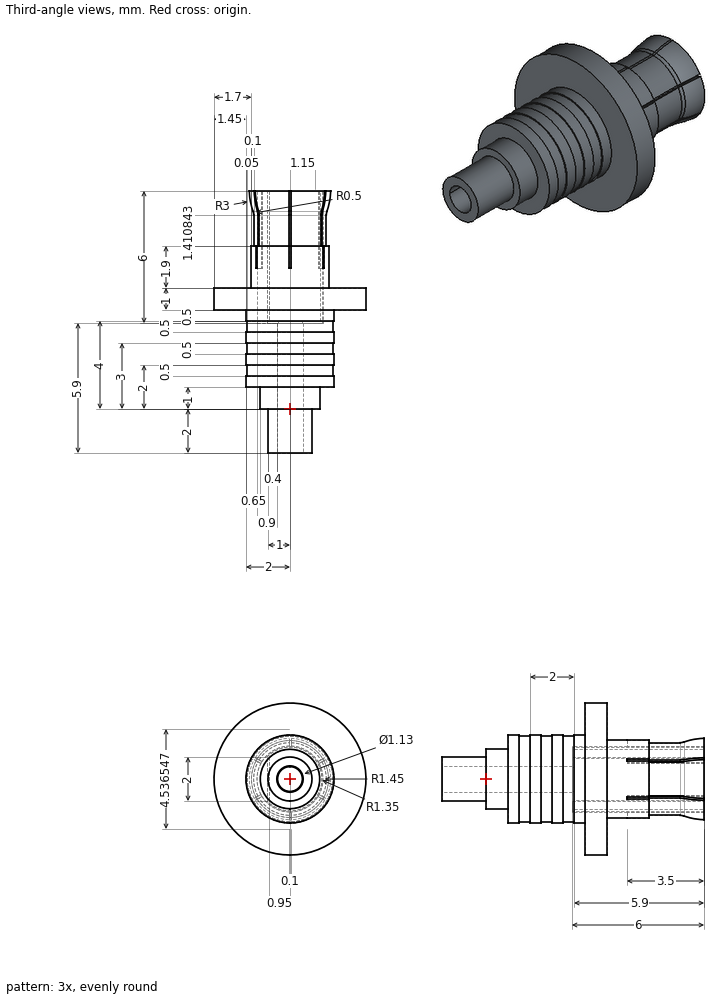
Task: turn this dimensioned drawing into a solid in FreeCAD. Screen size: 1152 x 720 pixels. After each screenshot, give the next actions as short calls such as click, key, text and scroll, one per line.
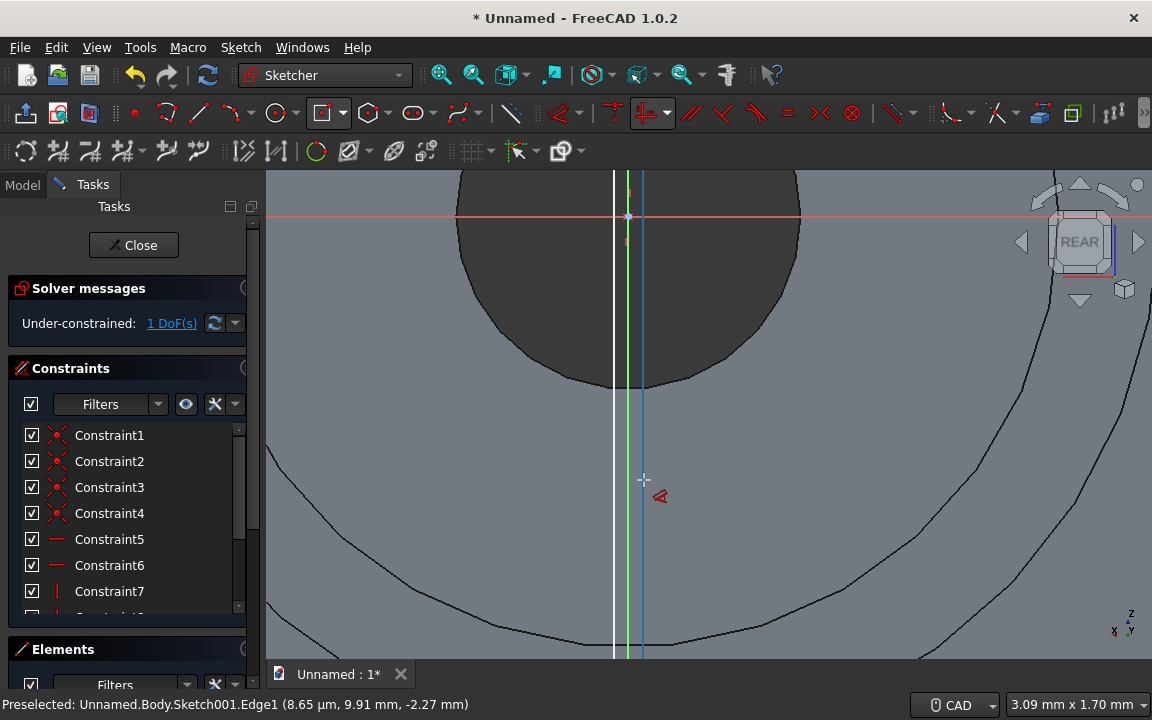
click(643, 477)
click(677, 414)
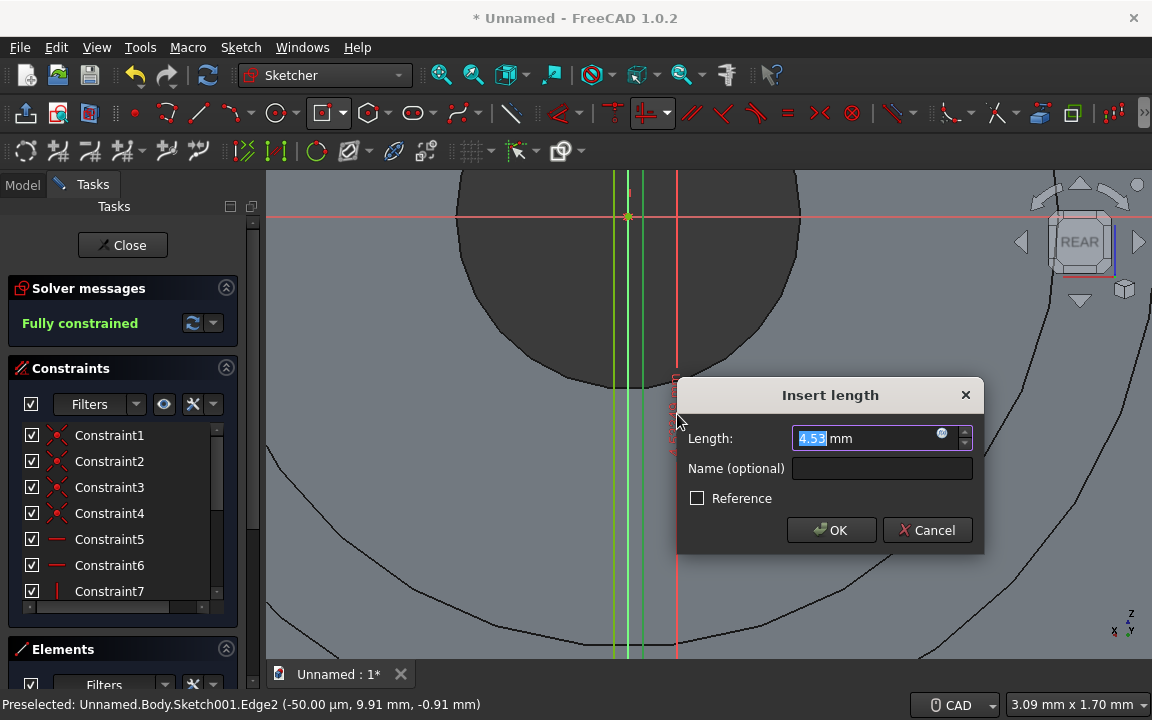
text(4.536547)
key(Return)
key(Escape)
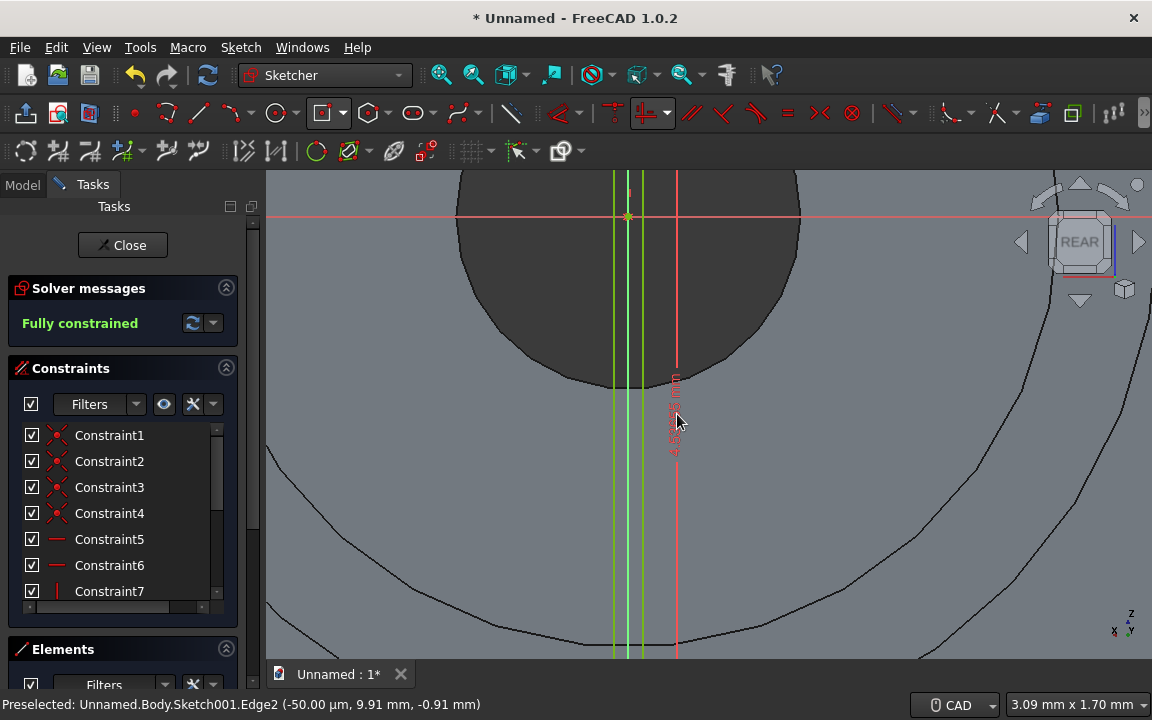
click(123, 245)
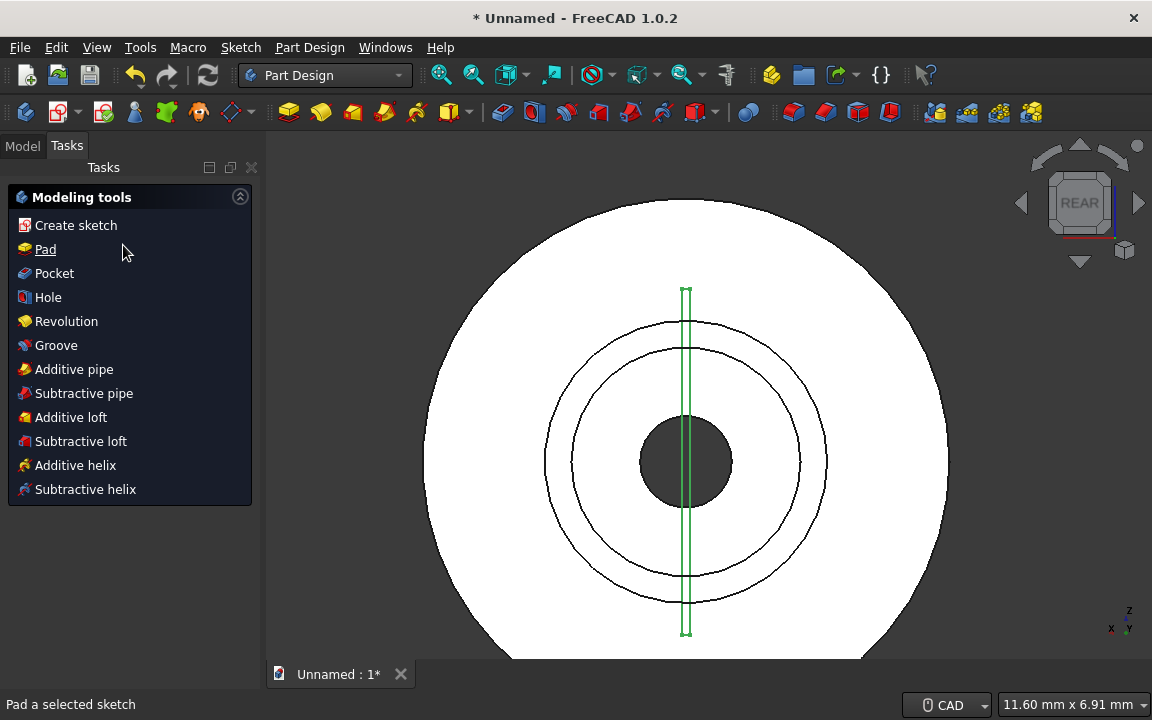
click(504, 112)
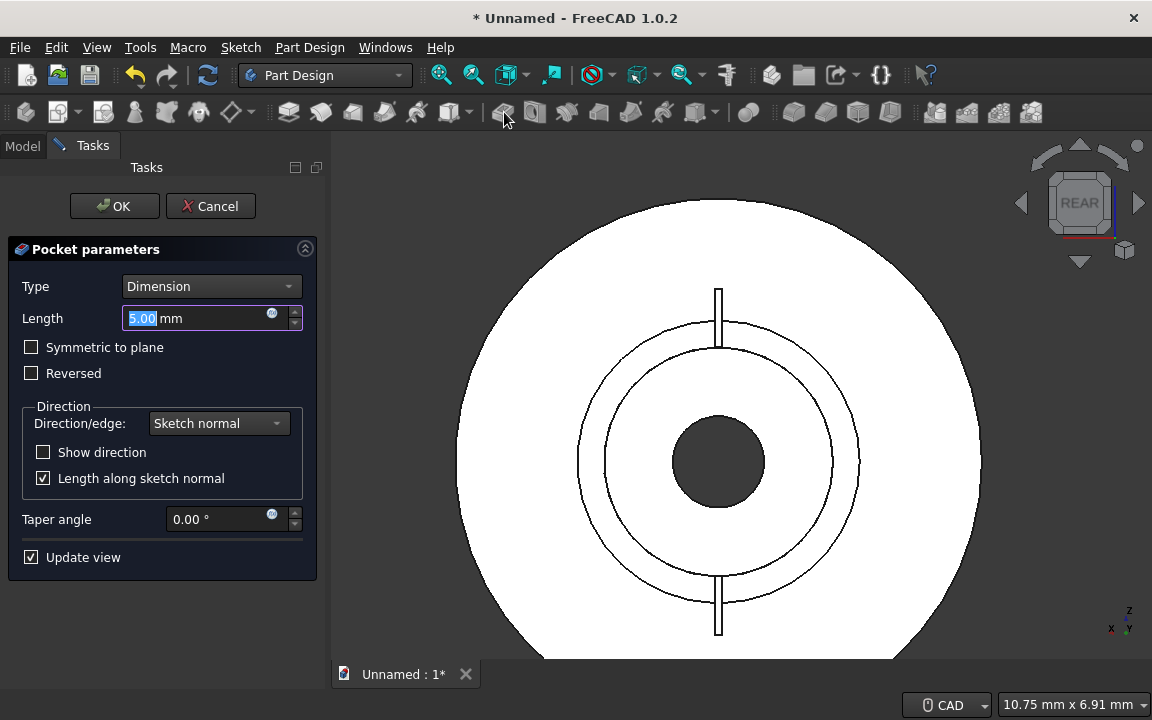
text(3.5)
key(Tab)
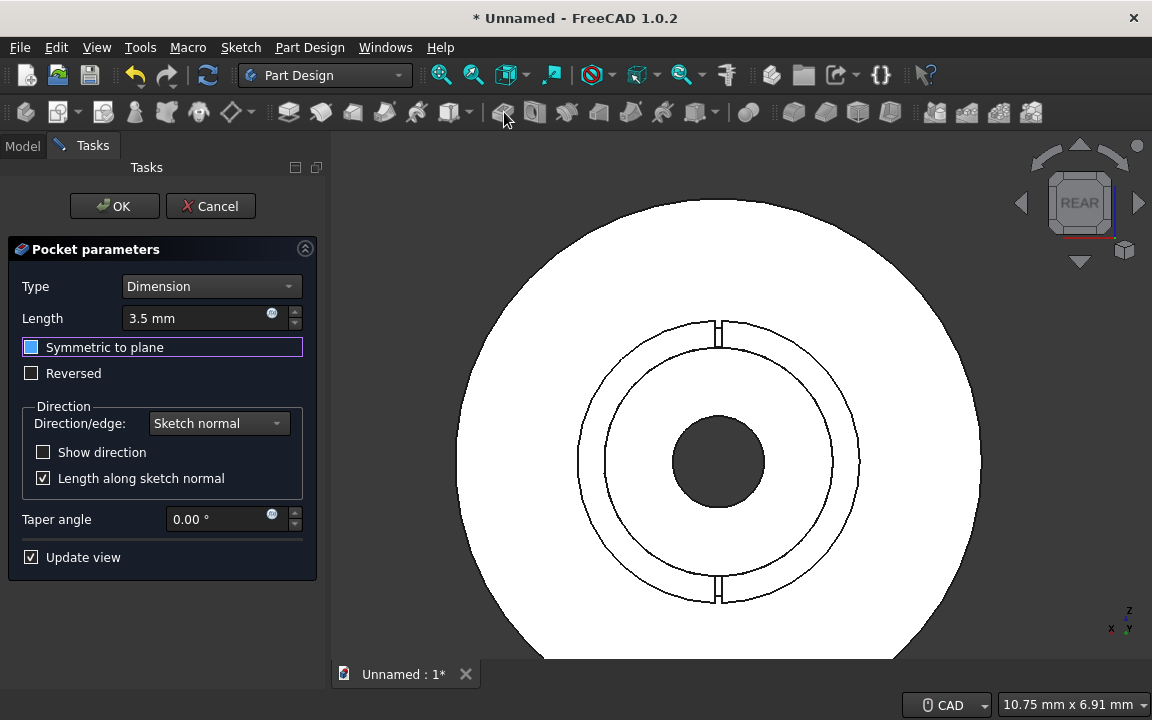
click(115, 206)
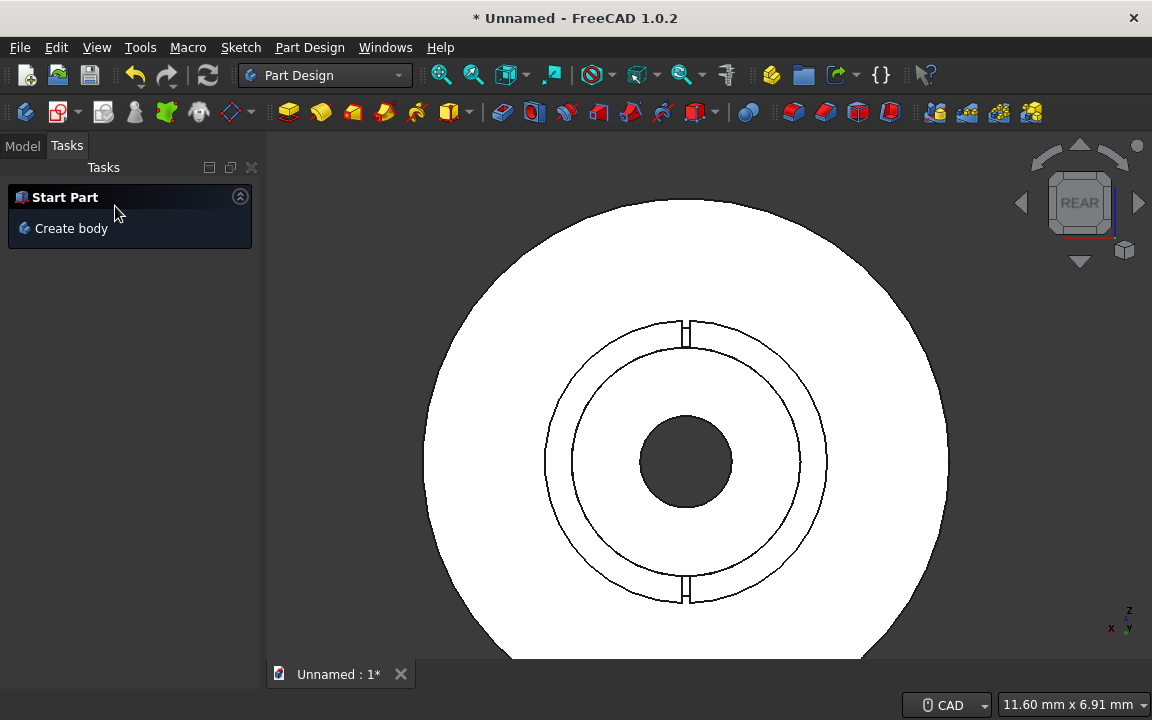
click(442, 76)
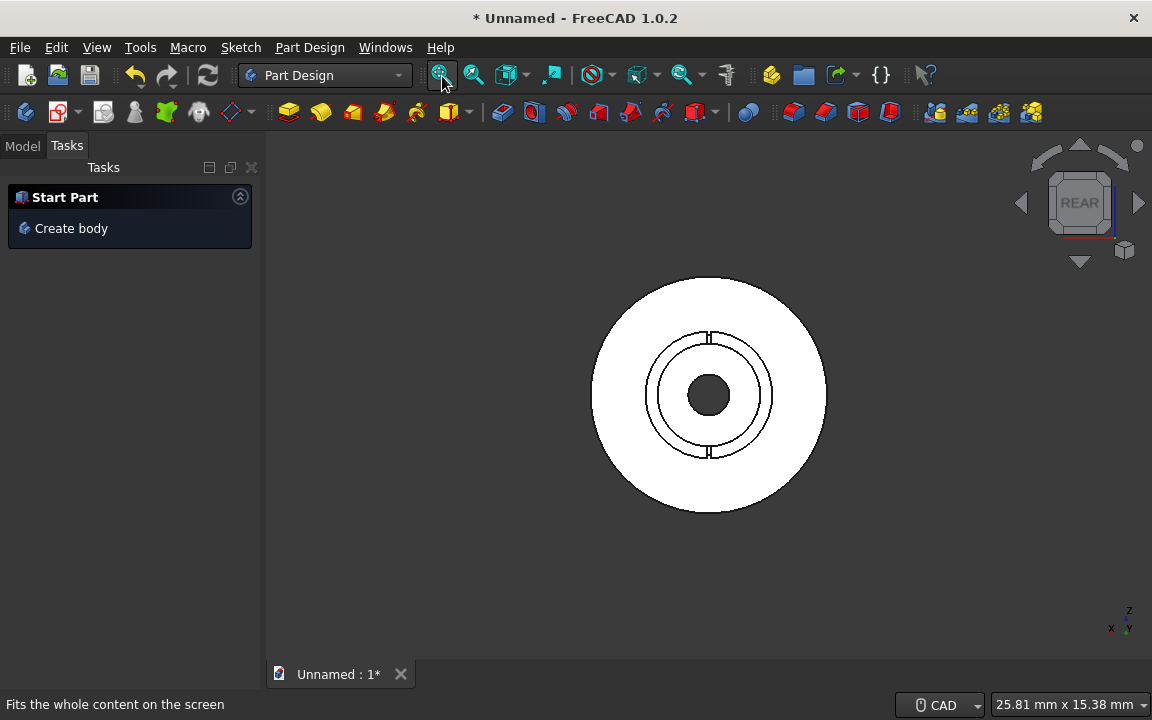
click(23, 145)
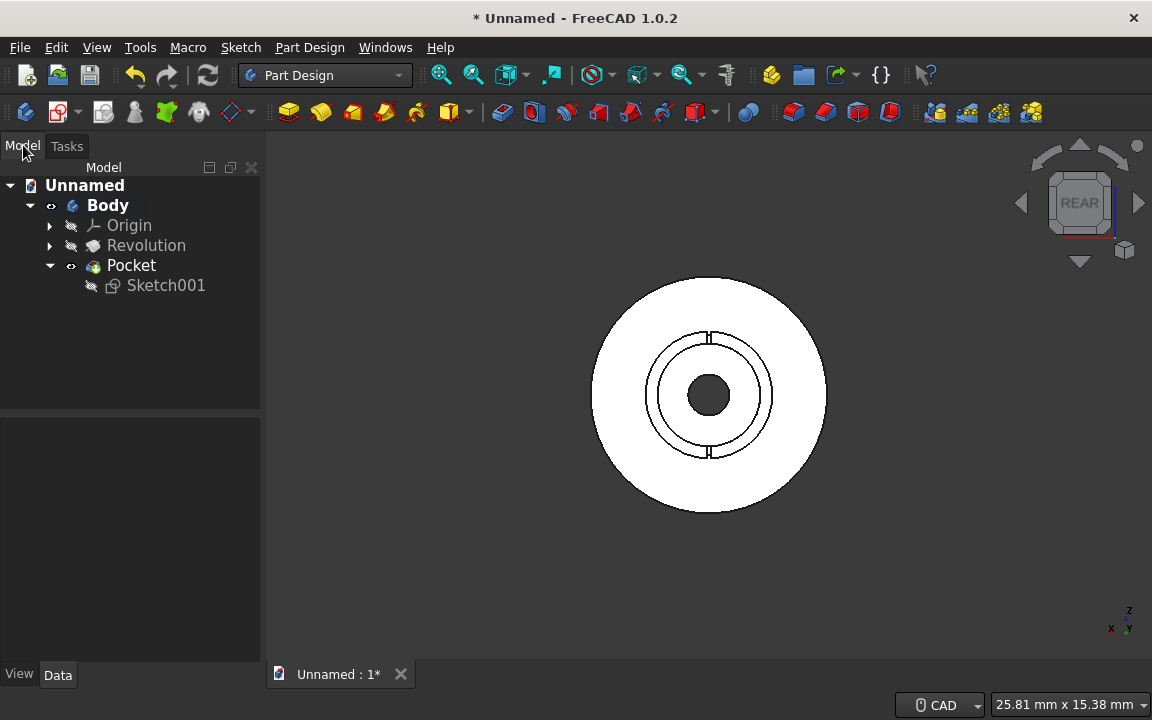
click(116, 266)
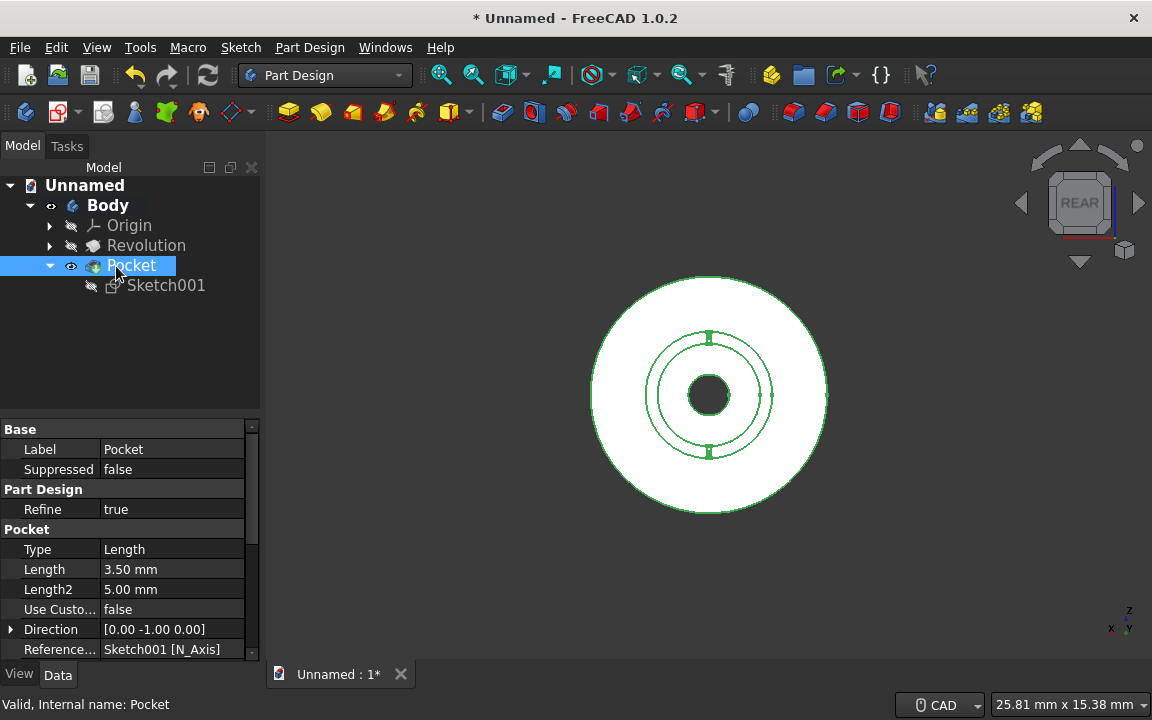
click(1000, 112)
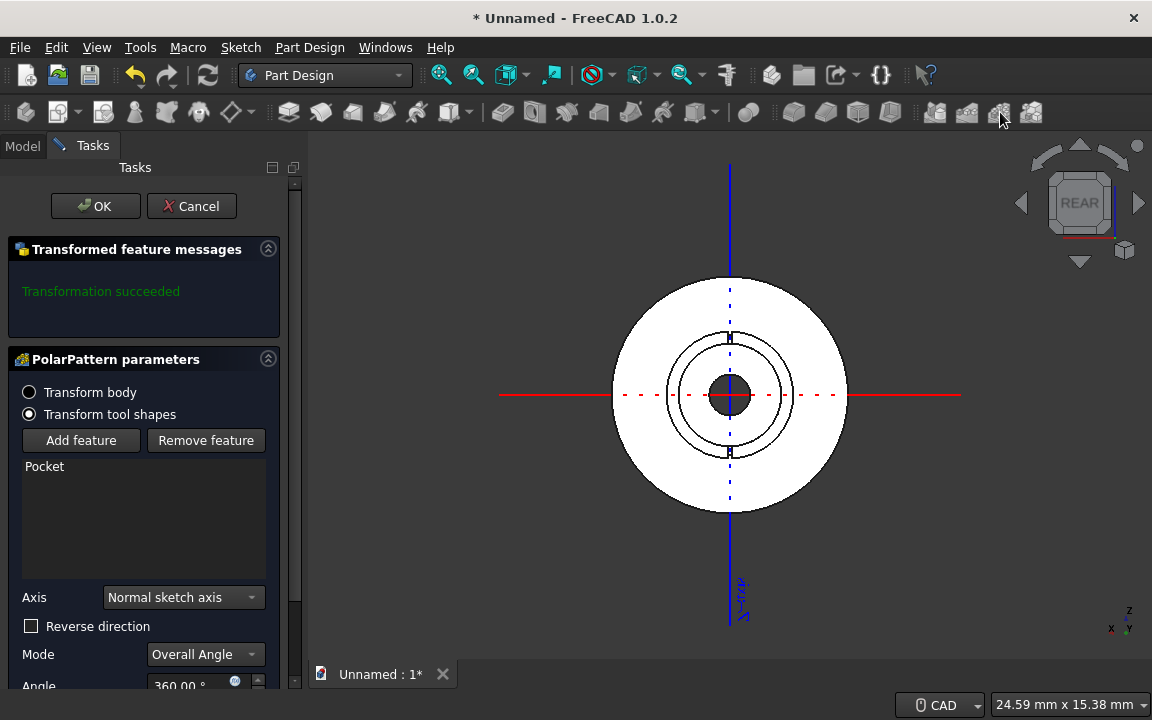
click(184, 598)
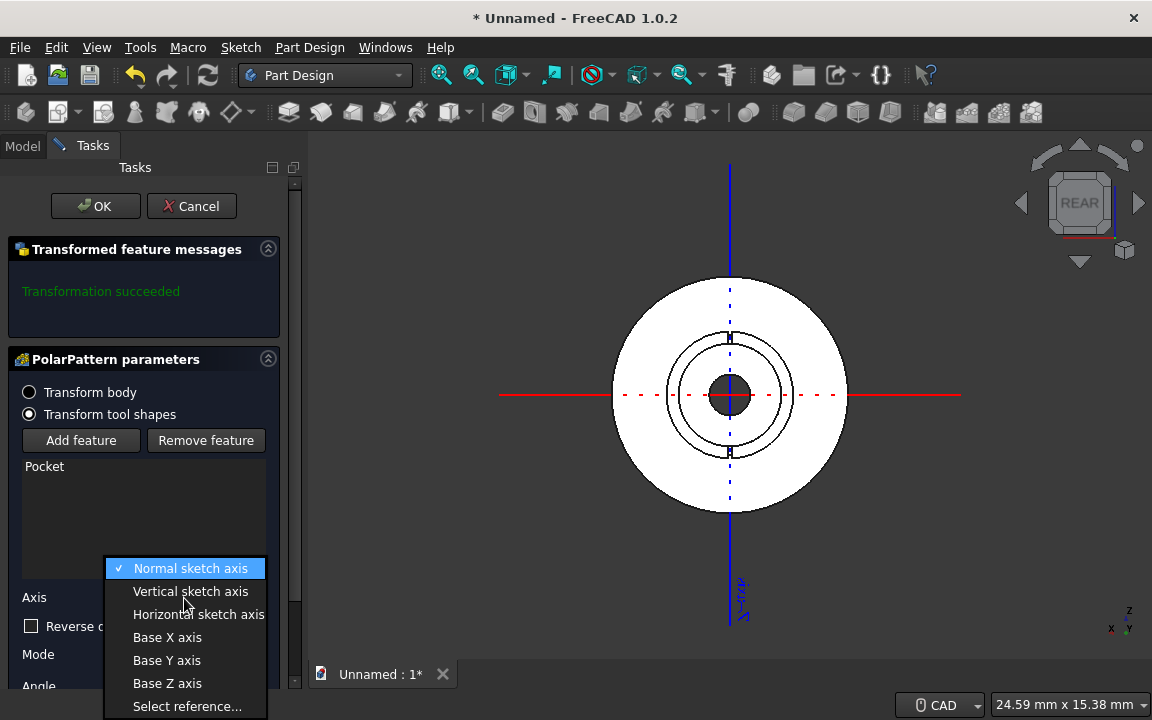
click(184, 660)